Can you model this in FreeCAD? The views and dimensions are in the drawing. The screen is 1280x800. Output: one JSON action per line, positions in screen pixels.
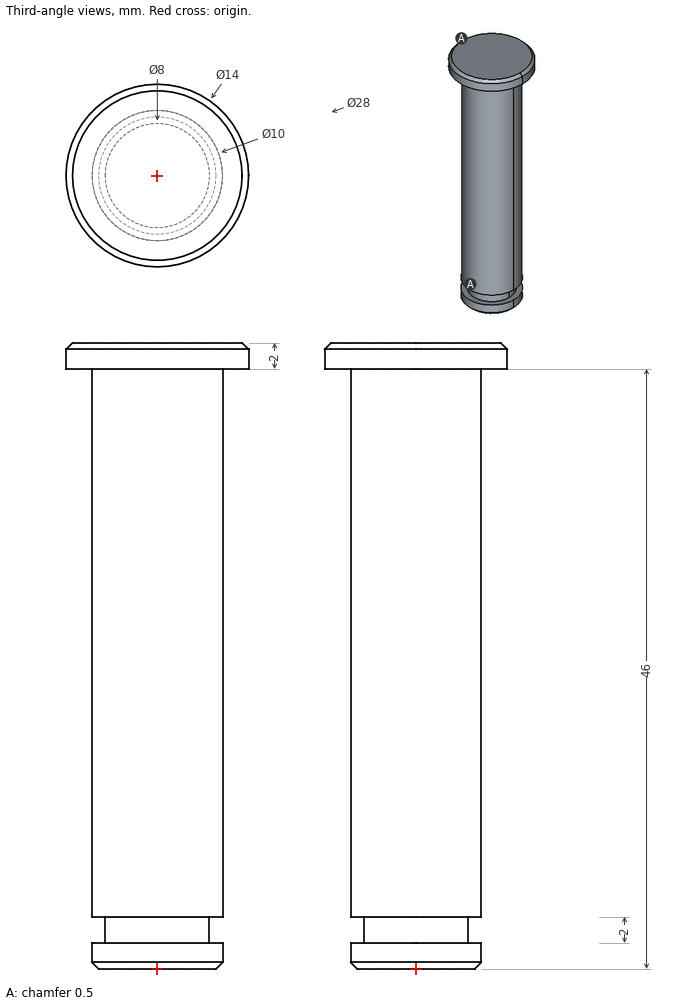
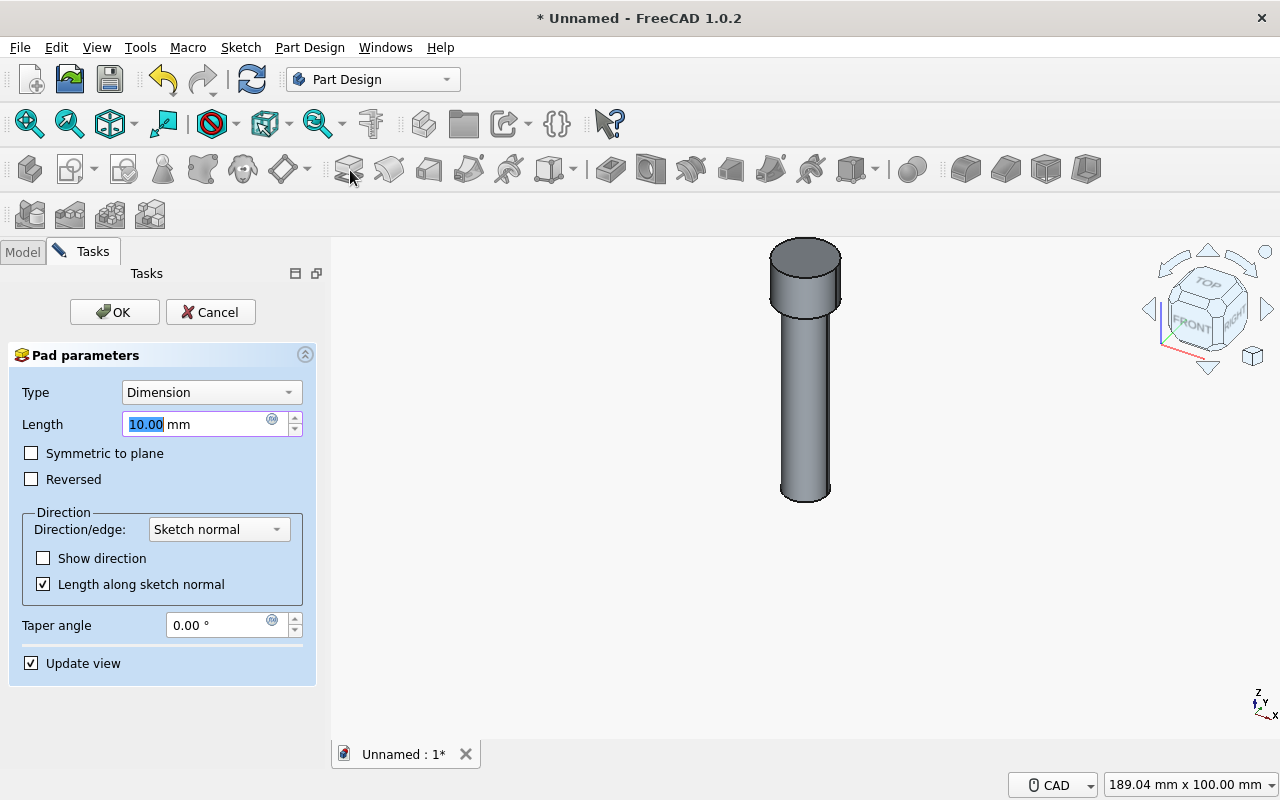
{"action": "type", "text": "2"}
{"action": "key", "text": "Tab"}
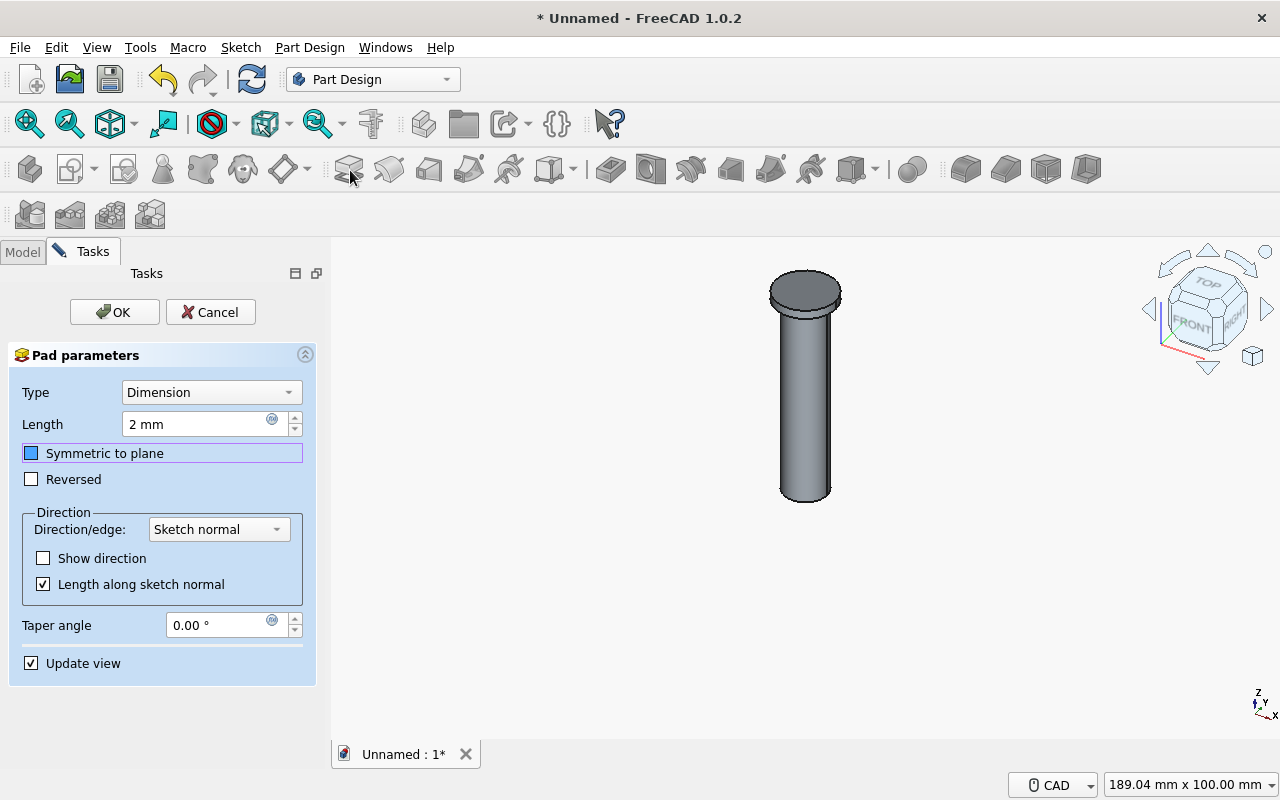
{"action": "left_click", "coordinate": [115, 312]}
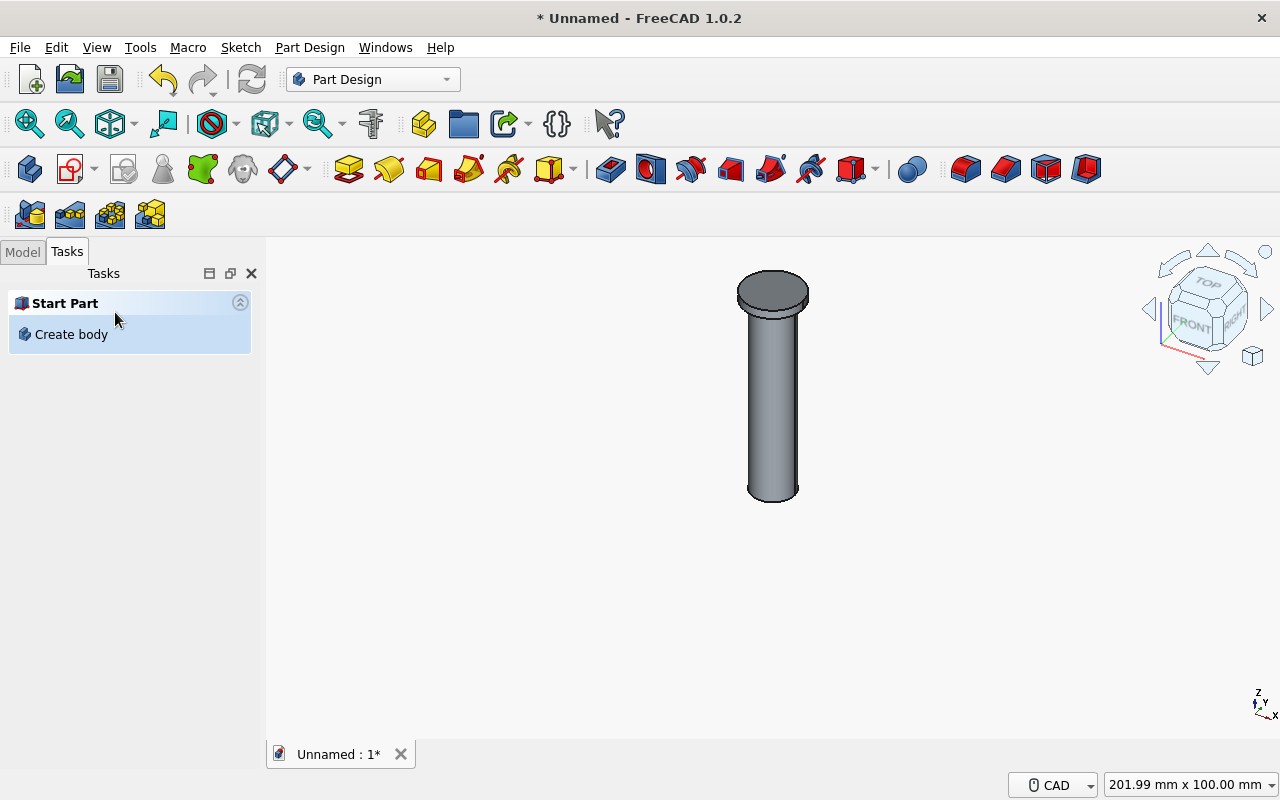
{"action": "left_click", "coordinate": [754, 497]}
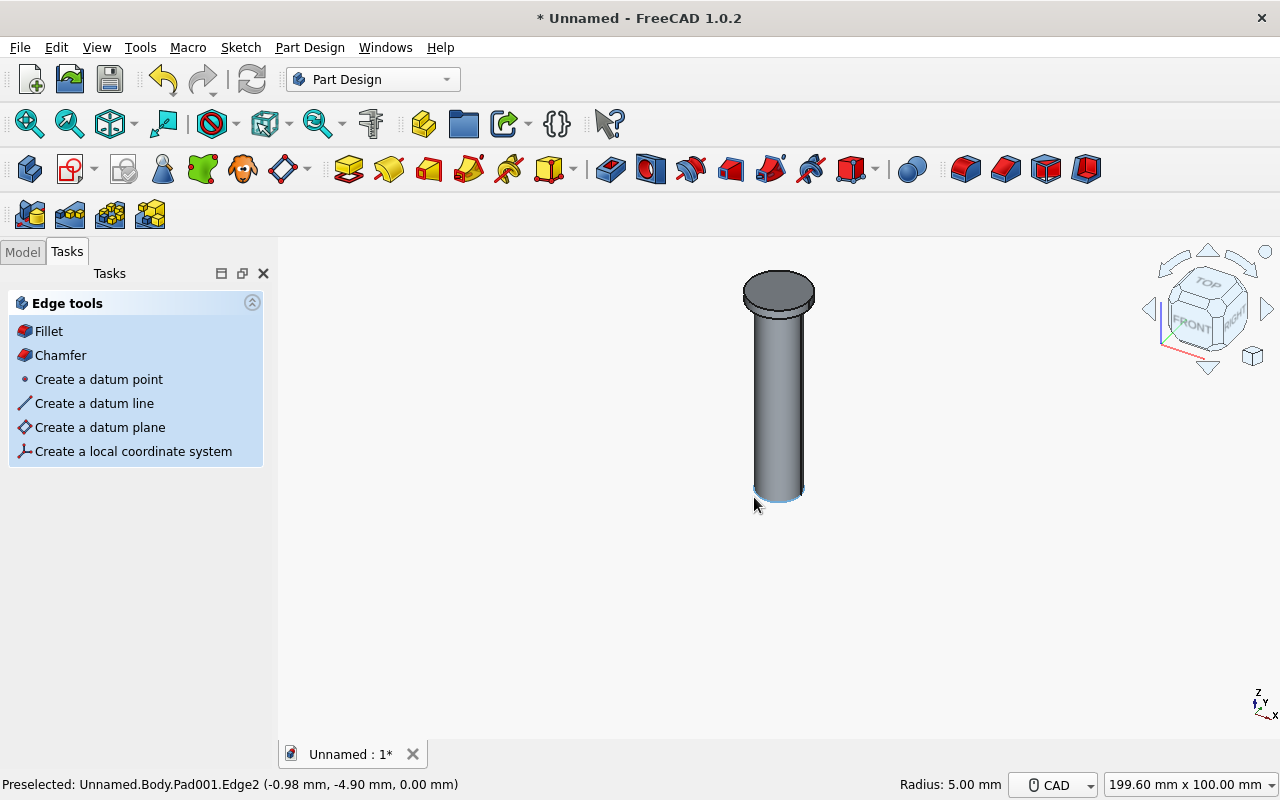
{"action": "left_click", "coordinate": [744, 292], "text": "ctrl"}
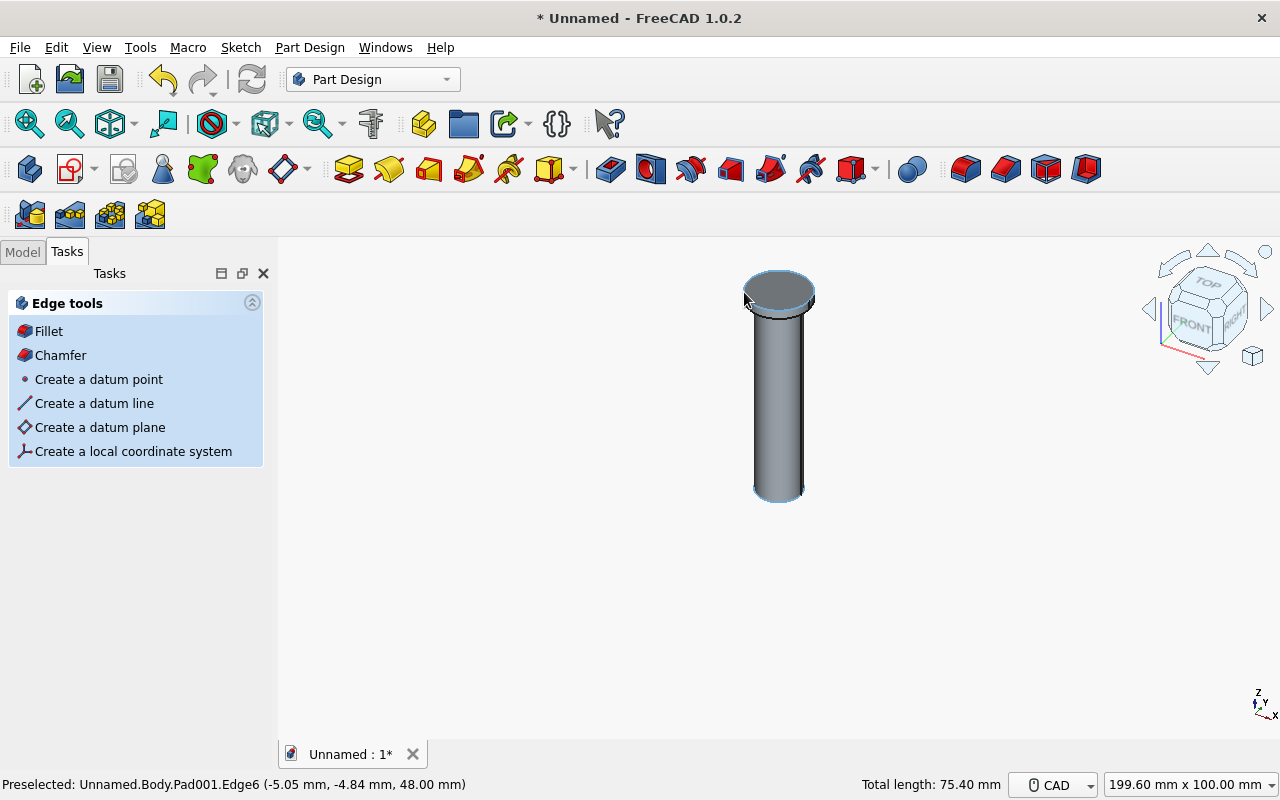
{"action": "left_click", "coordinate": [1006, 170]}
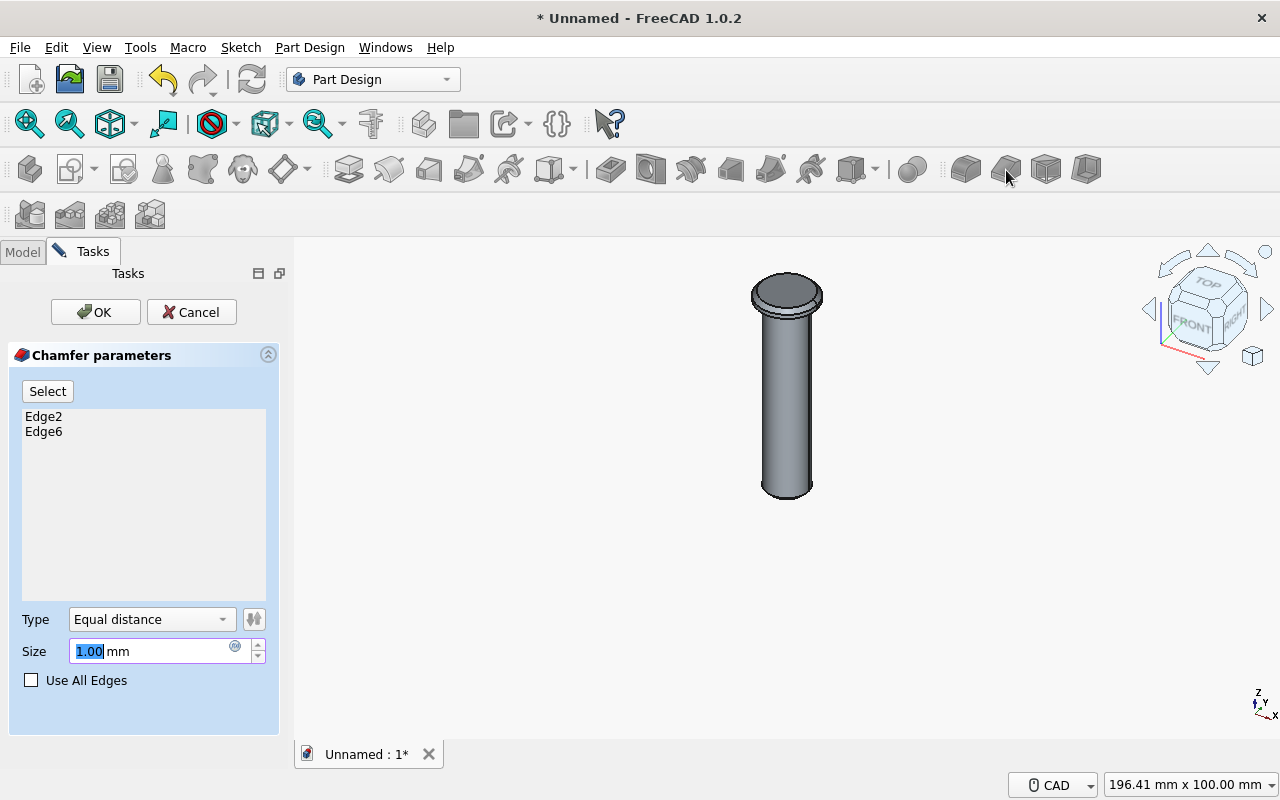
{"action": "type", "text": "0.5"}
{"action": "key", "text": "Tab"}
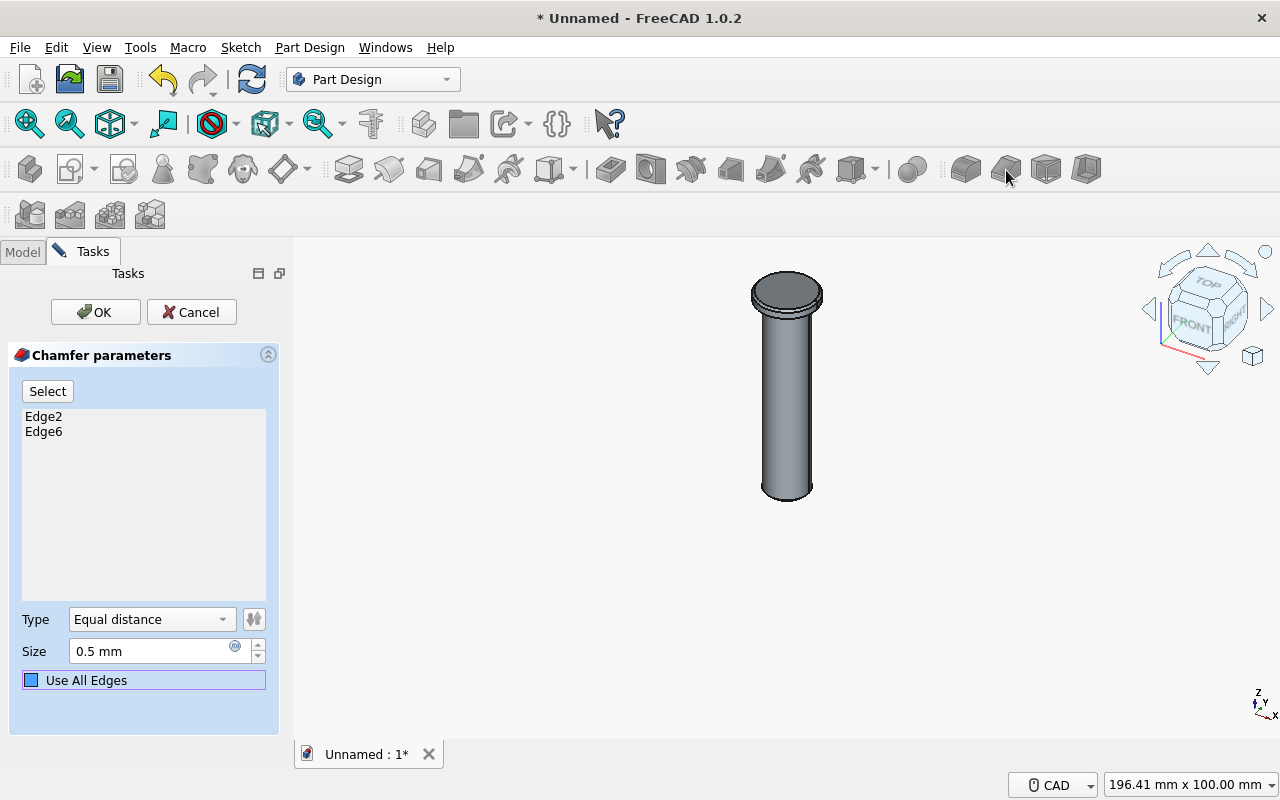
{"action": "left_click", "coordinate": [96, 312]}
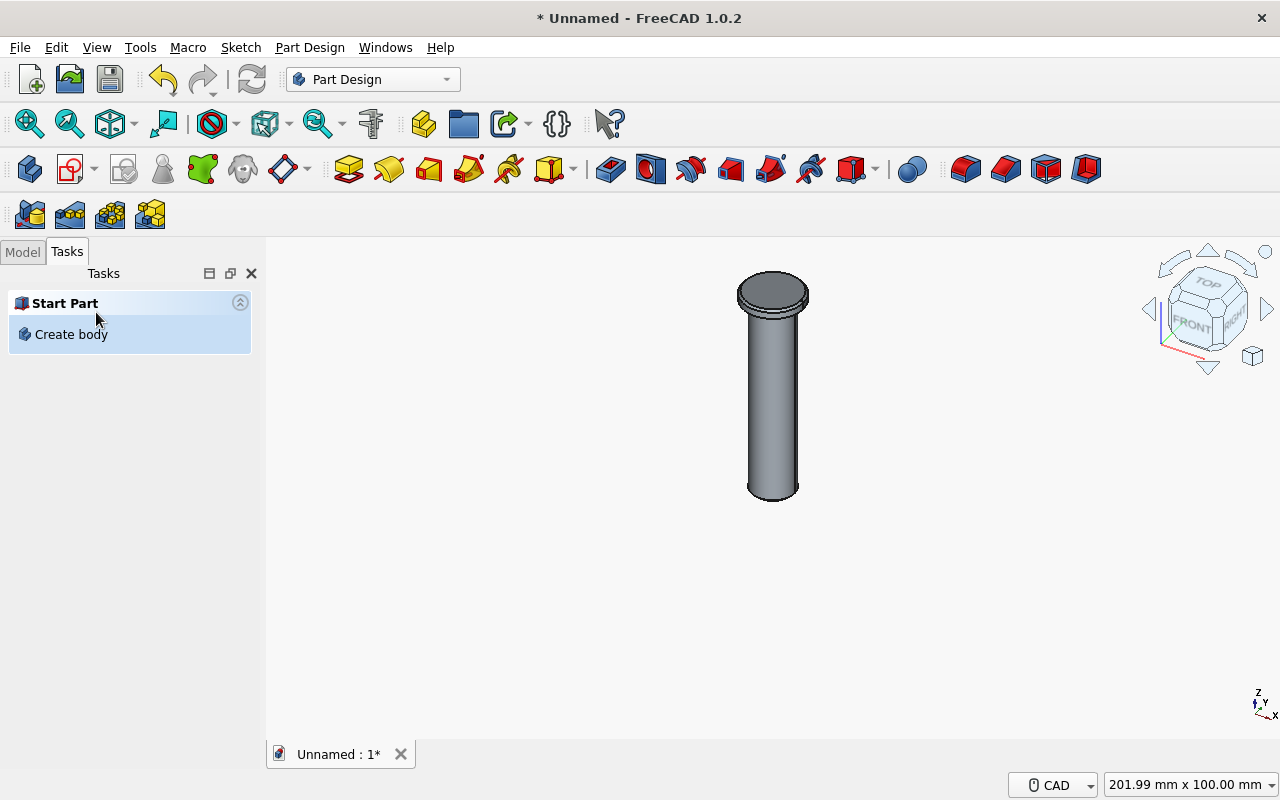
{"action": "left_click", "coordinate": [23, 251]}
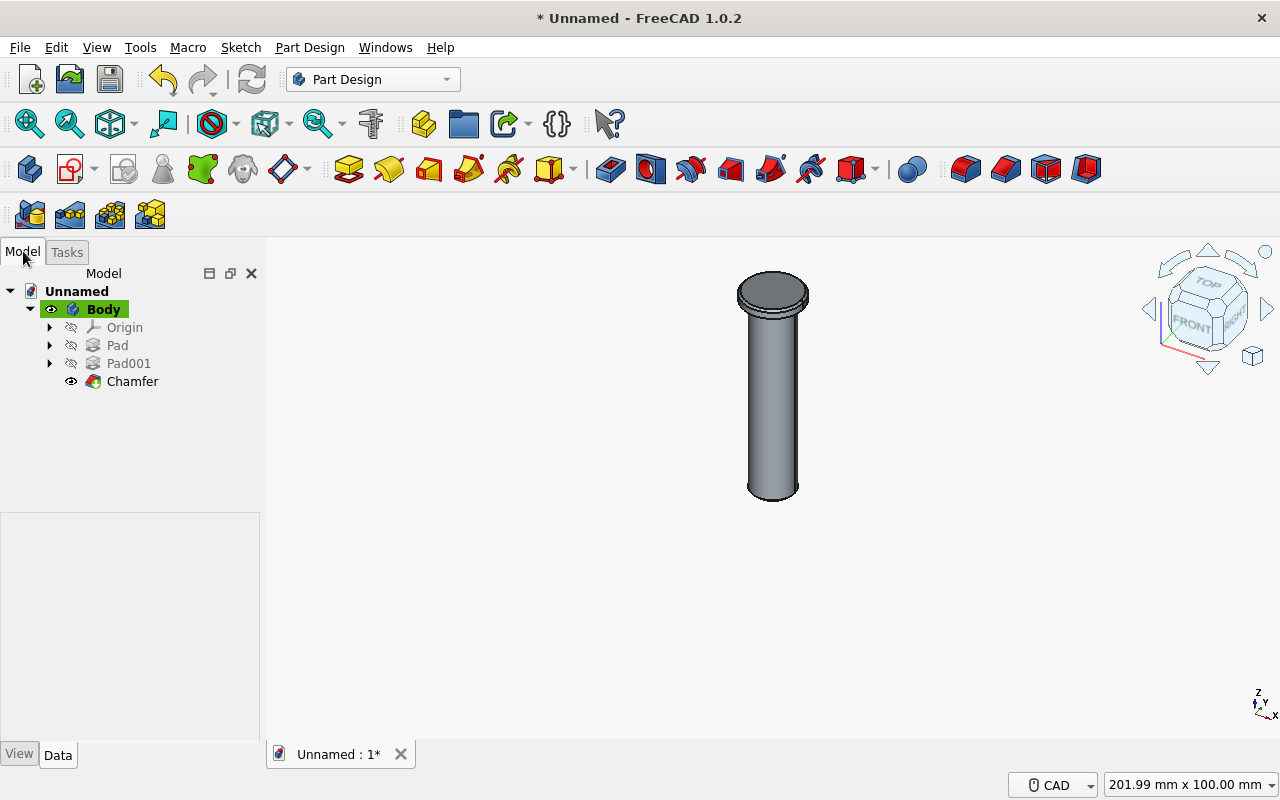
{"action": "left_click", "coordinate": [50, 327]}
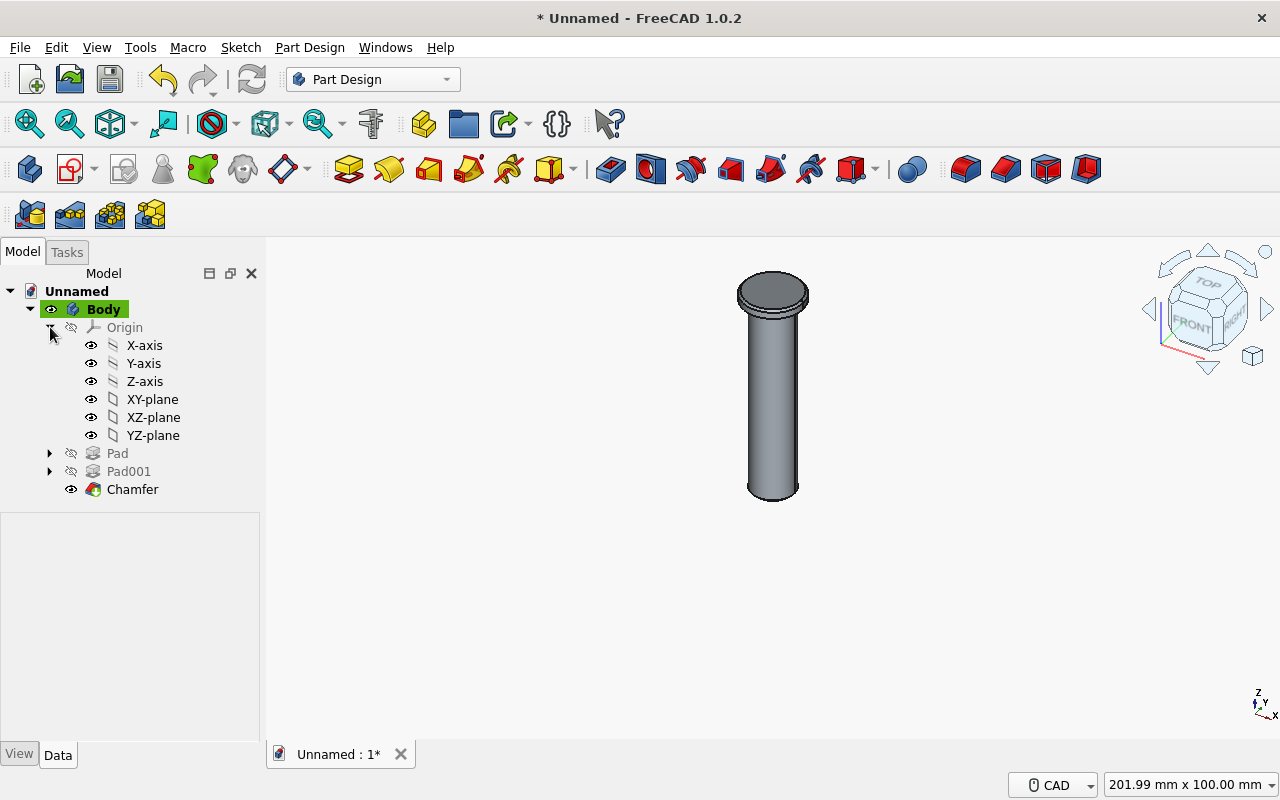
{"action": "left_click", "coordinate": [136, 399]}